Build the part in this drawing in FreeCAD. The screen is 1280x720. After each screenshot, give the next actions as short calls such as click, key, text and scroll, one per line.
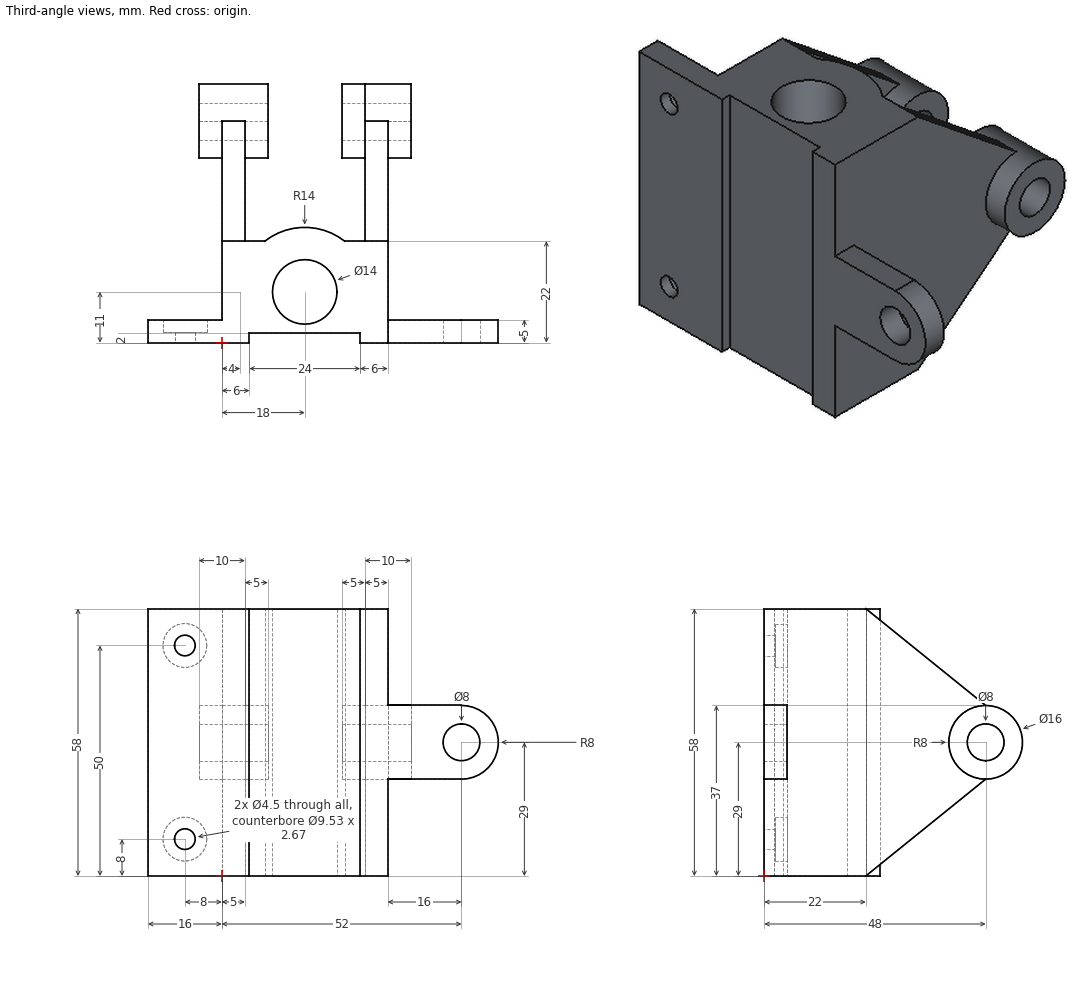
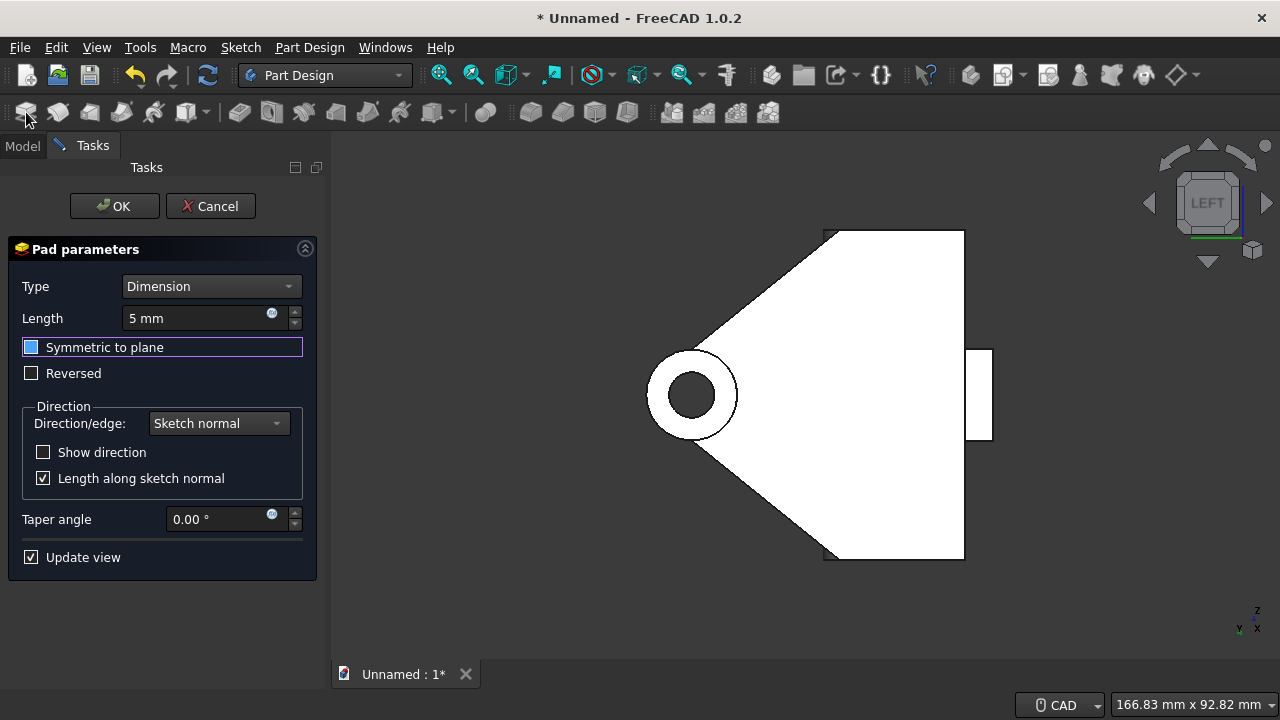
click(30, 373)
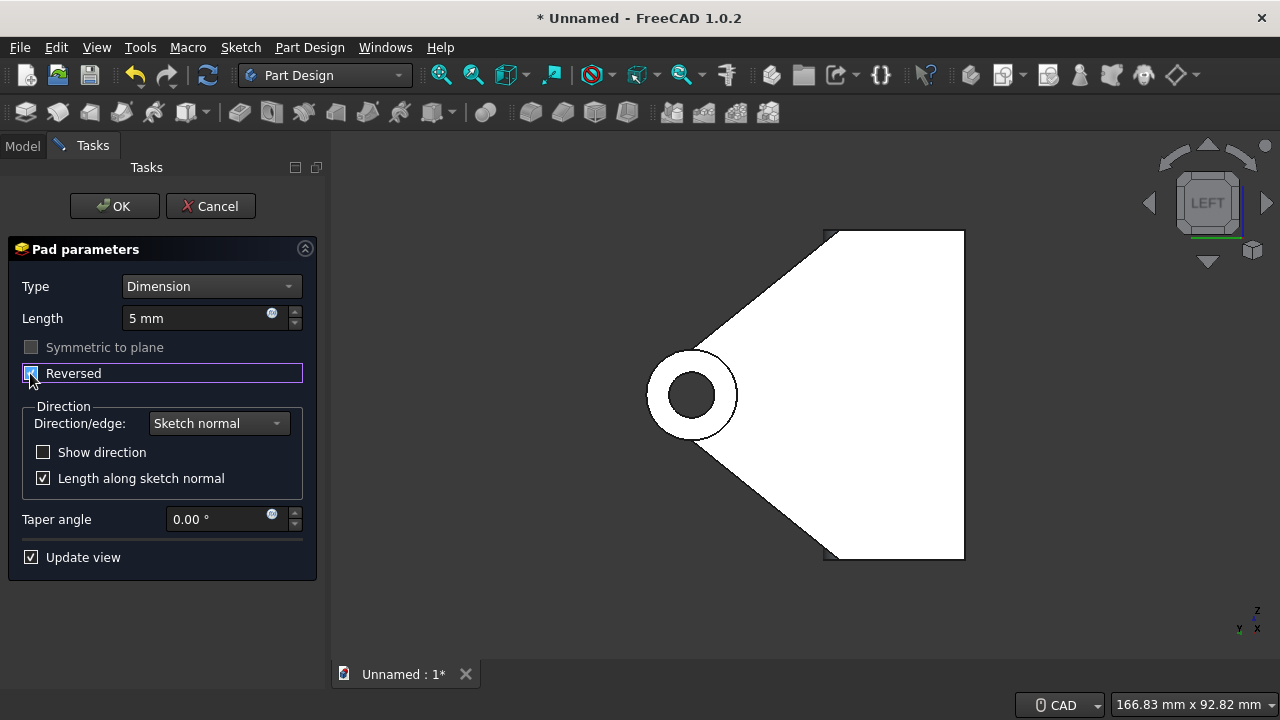
click(115, 206)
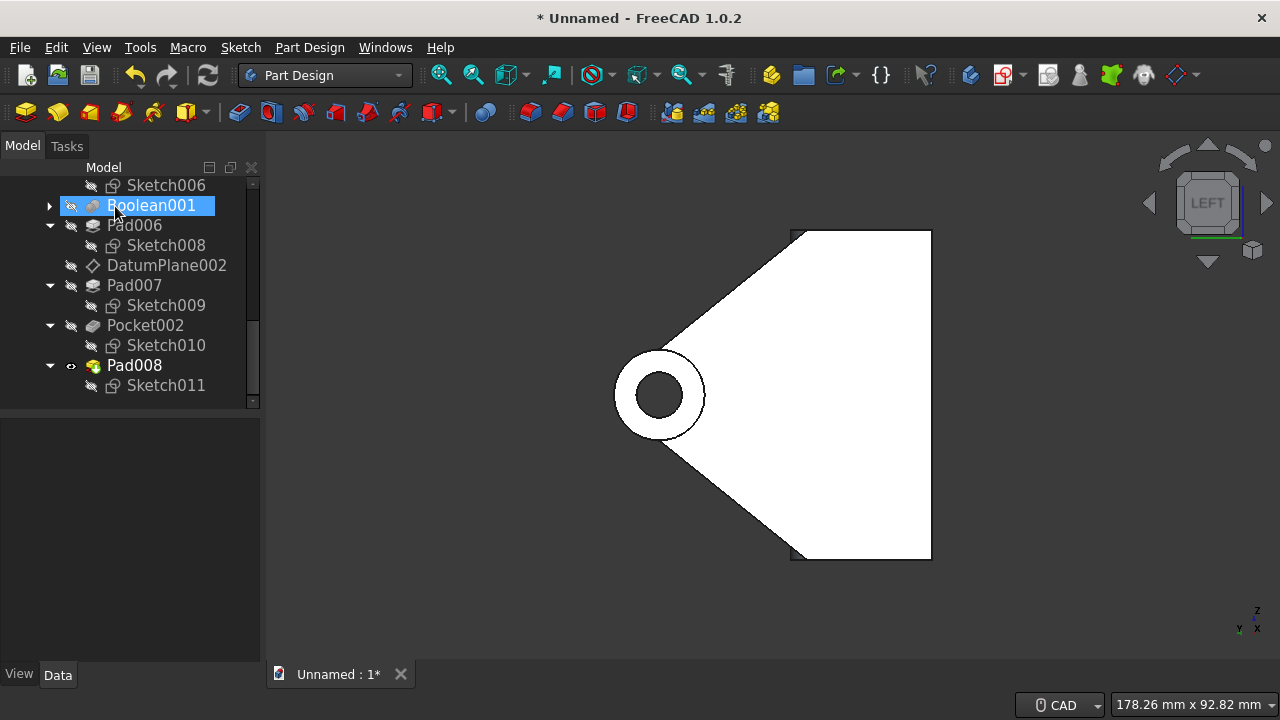
click(1004, 76)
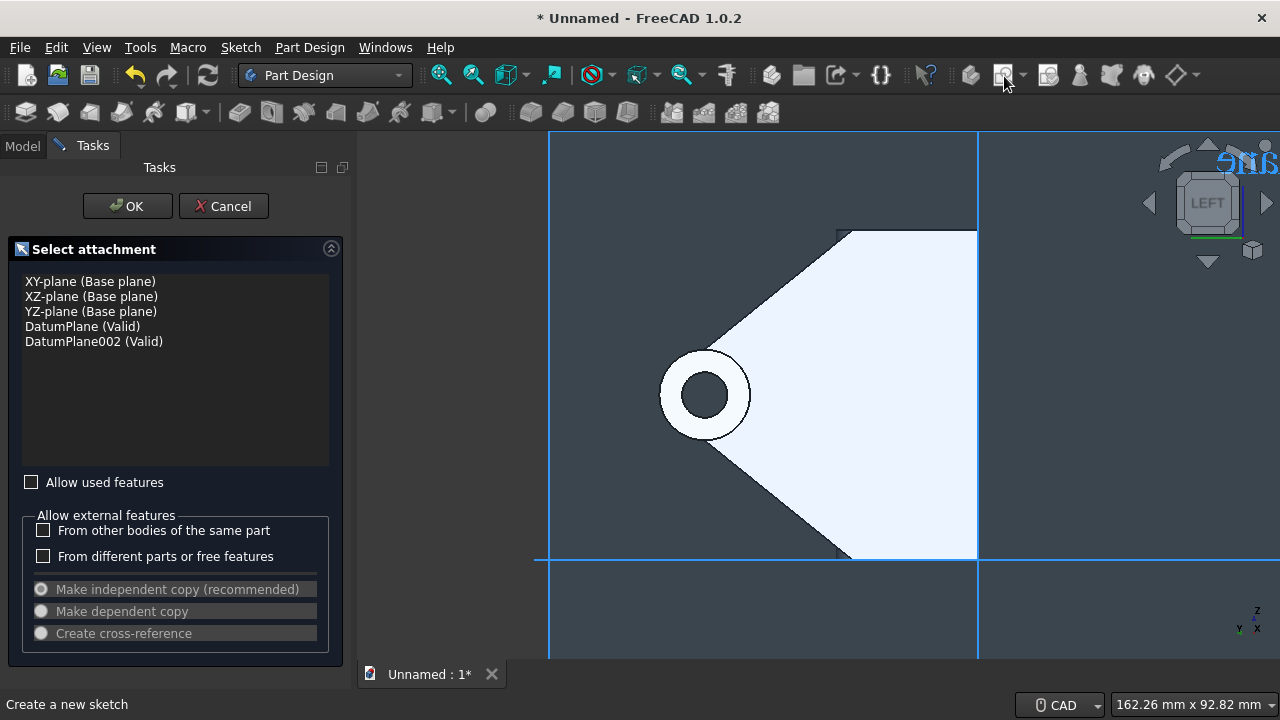
click(82, 296)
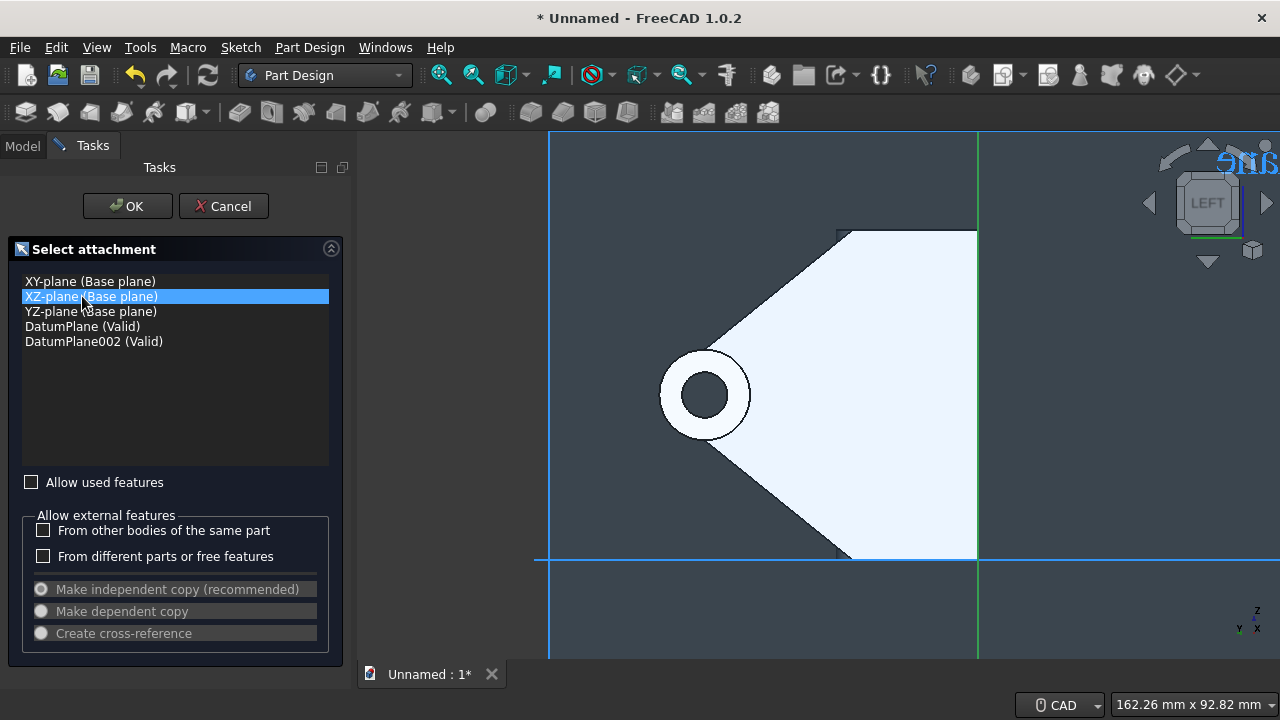
click(128, 206)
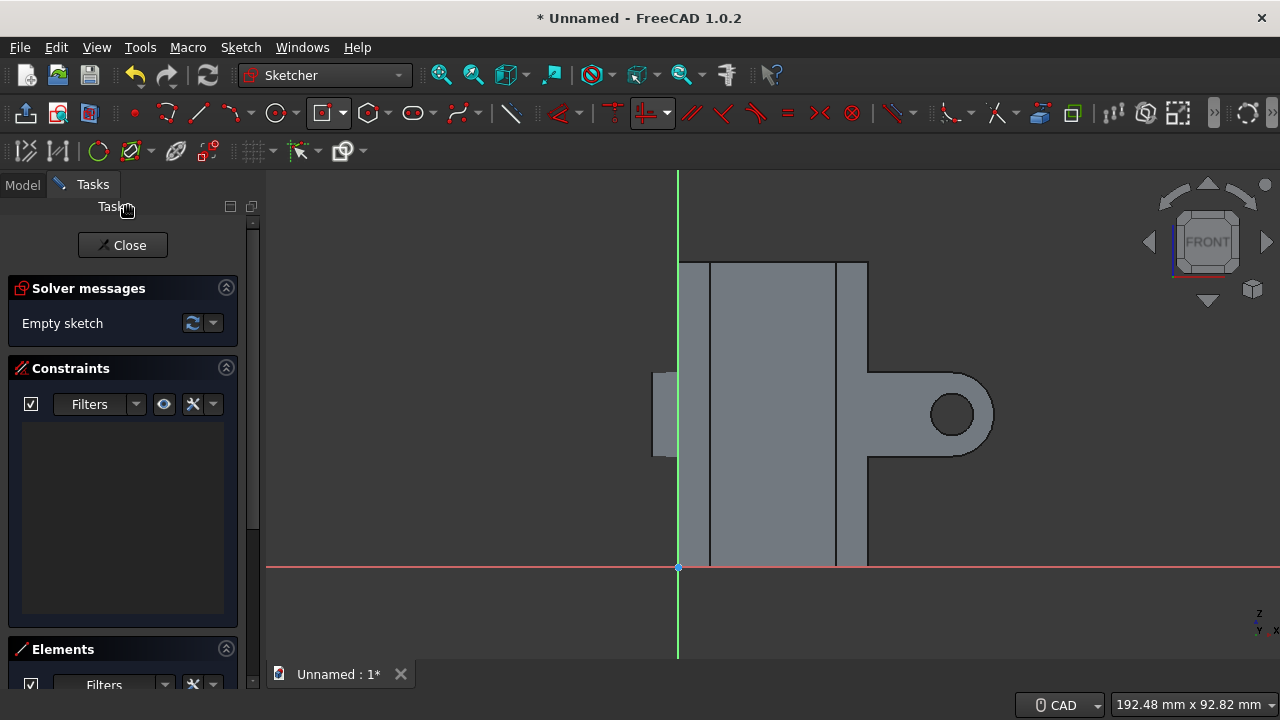
key(g)
key(r)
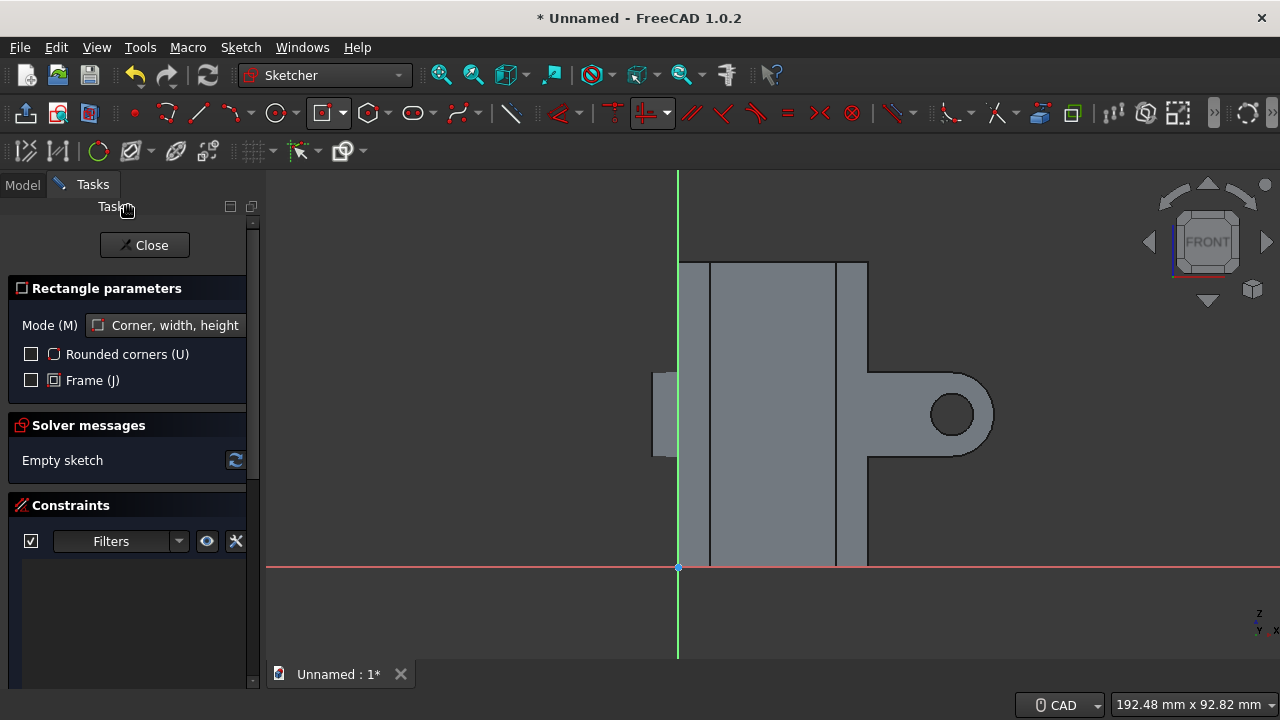
click(678, 567)
move(594, 262)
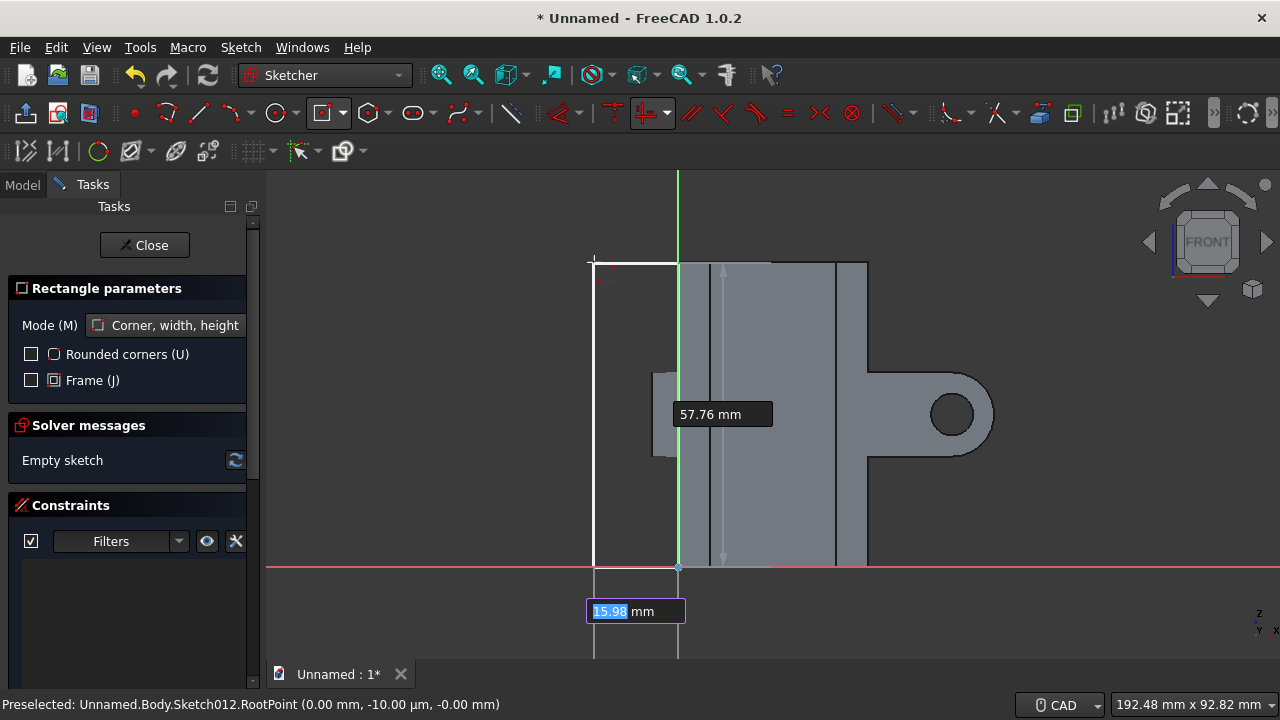
text(16)
key(Tab)
text(58)
key(Return)
key(Escape)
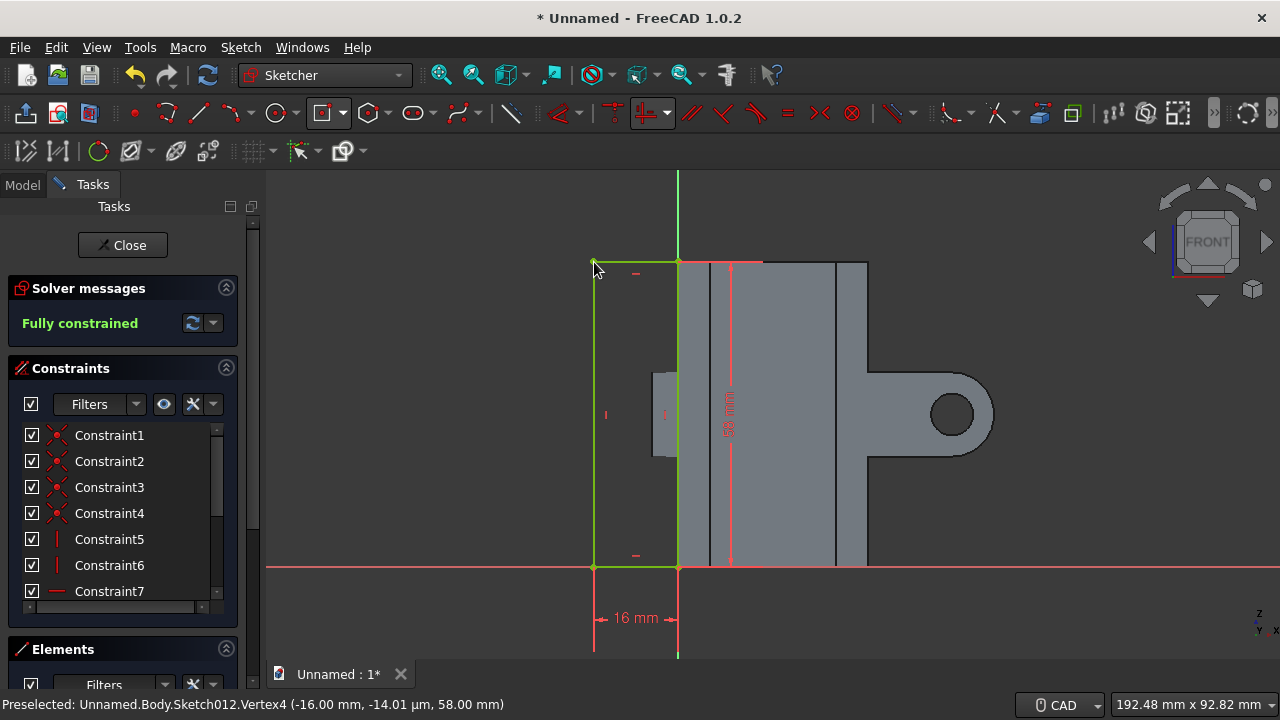
click(123, 245)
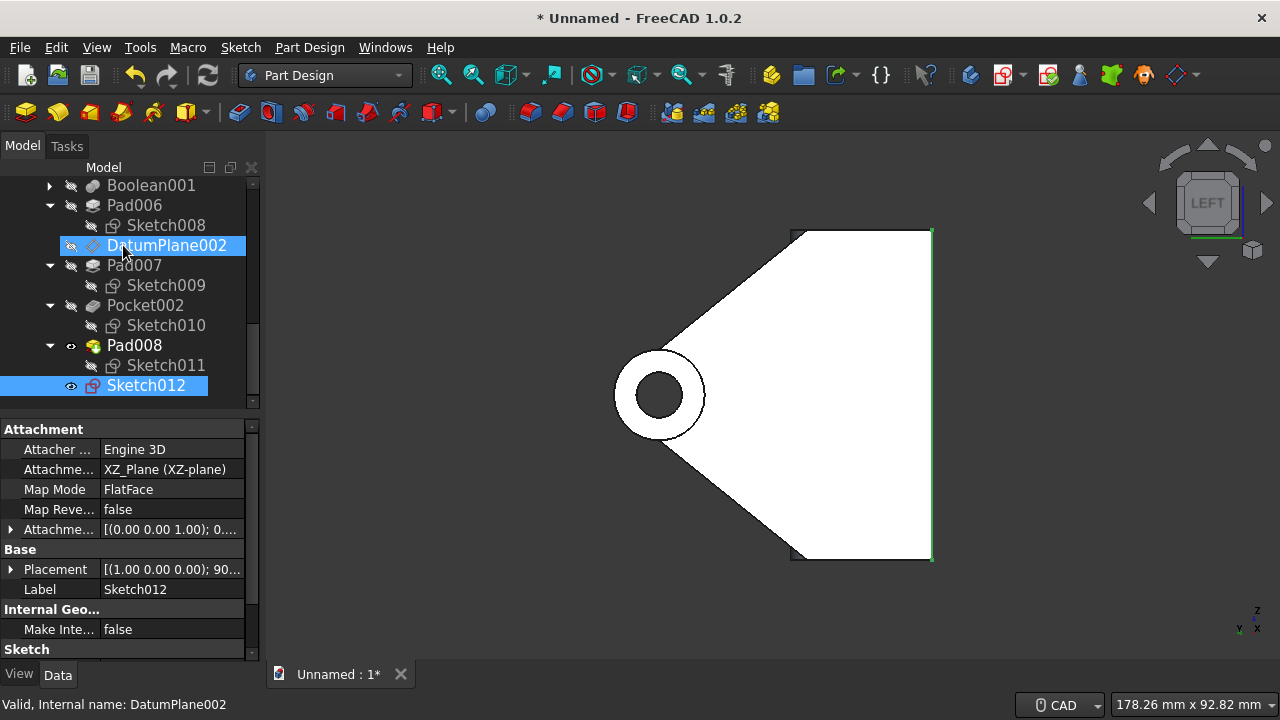
click(26, 112)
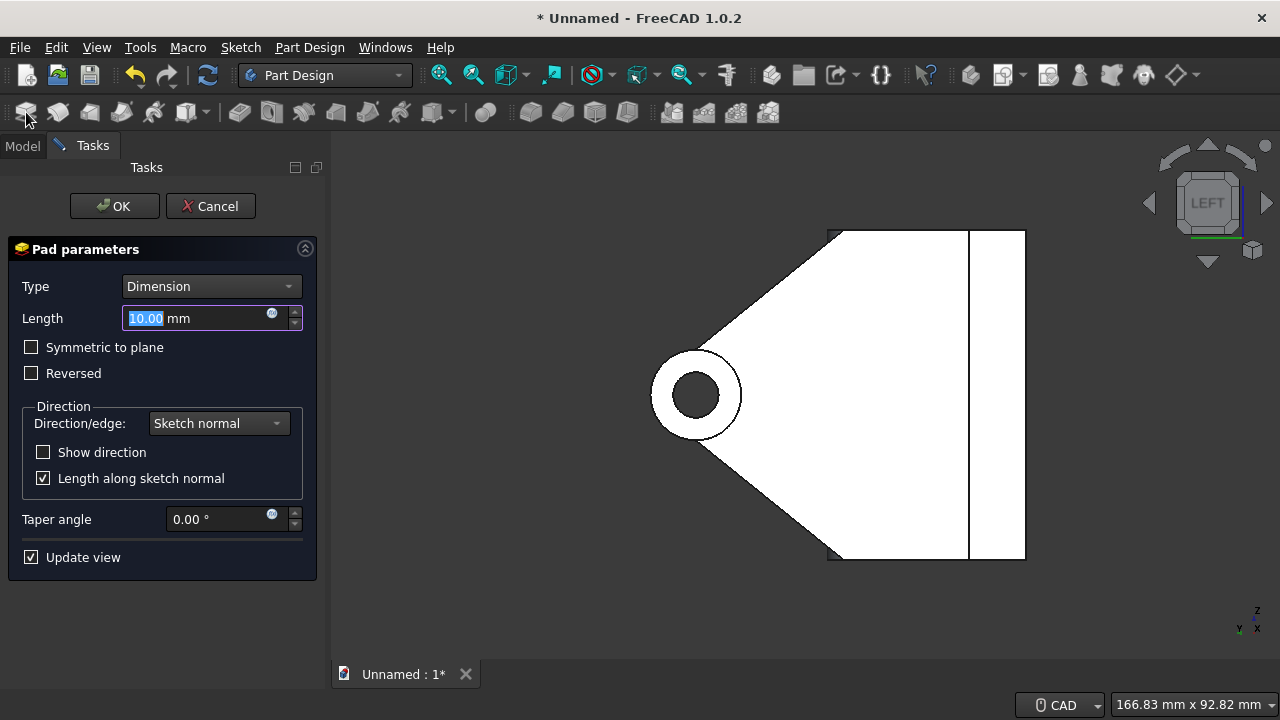
text(5)
key(Tab)